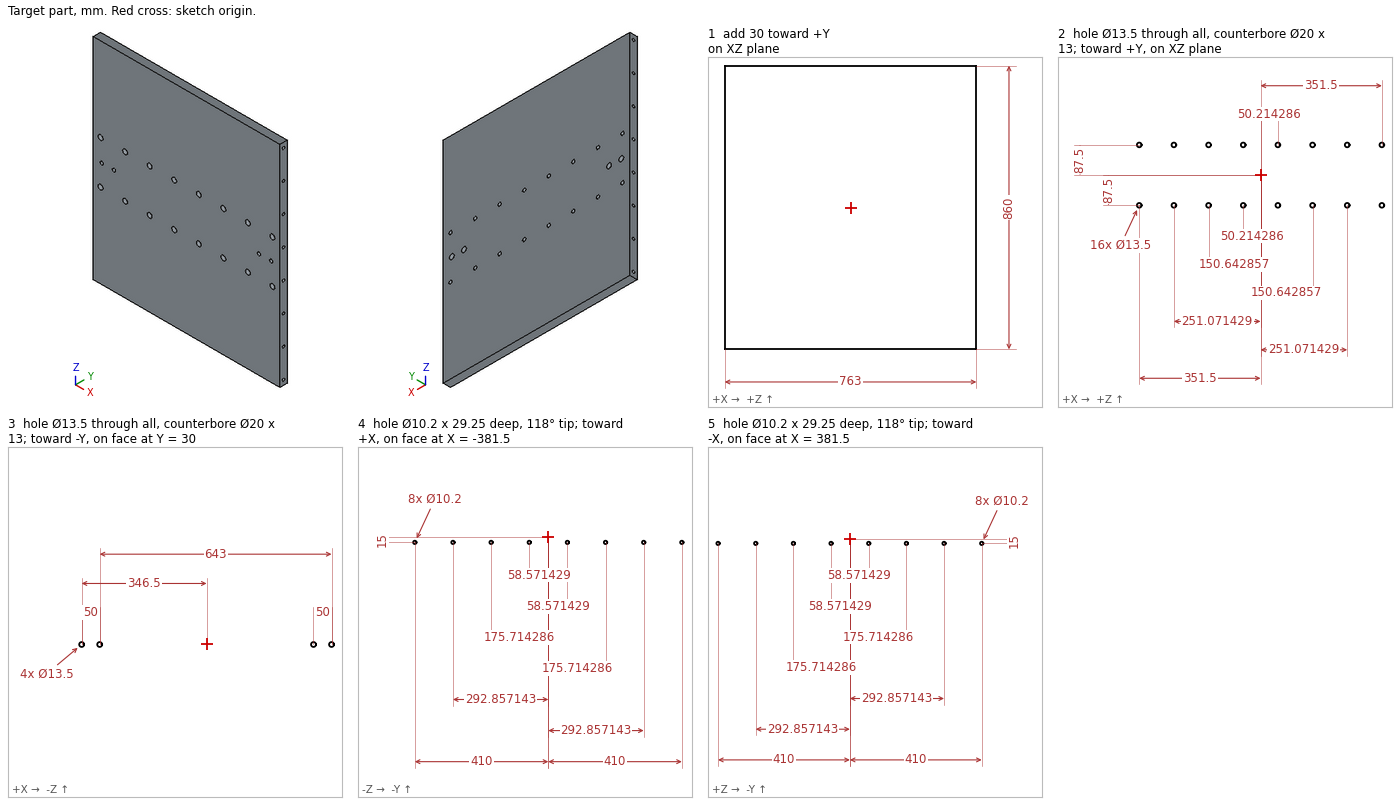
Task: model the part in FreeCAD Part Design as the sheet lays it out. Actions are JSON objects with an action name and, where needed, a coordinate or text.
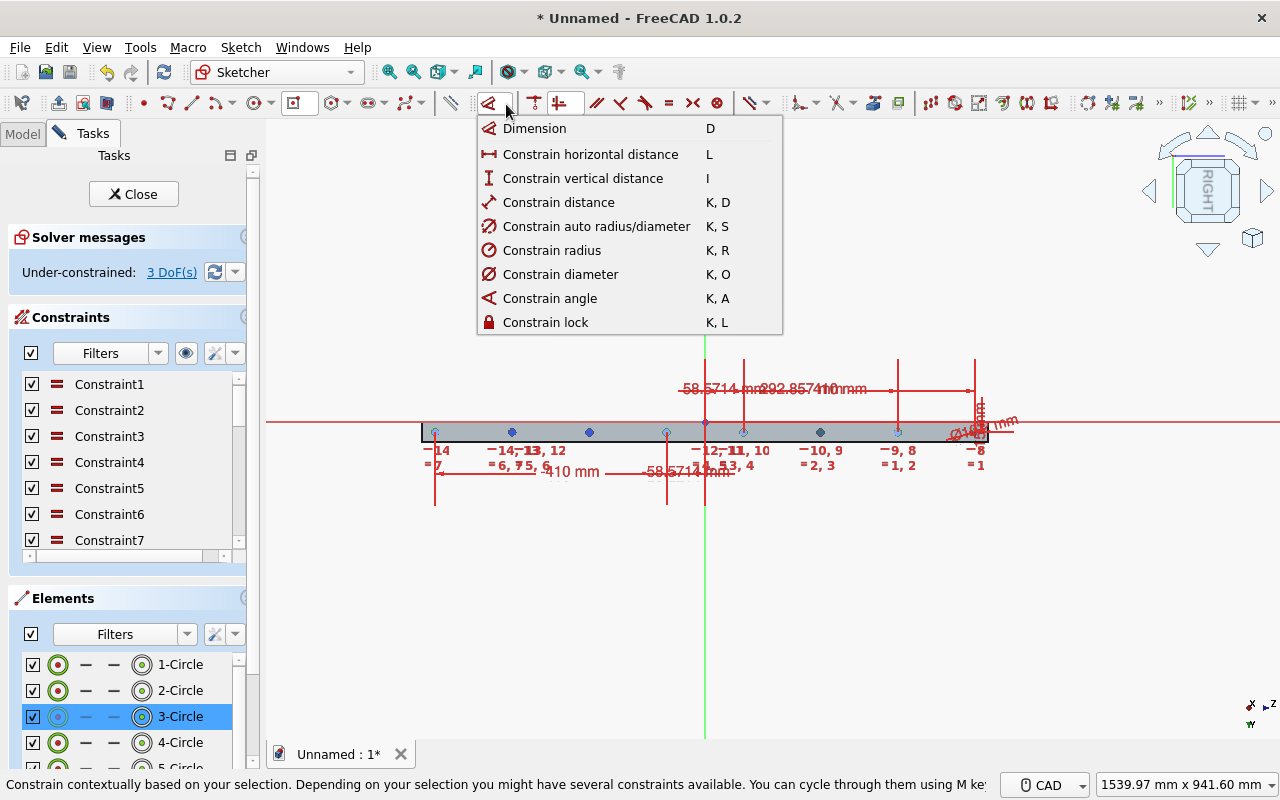
{"action": "left_click", "coordinate": [630, 154]}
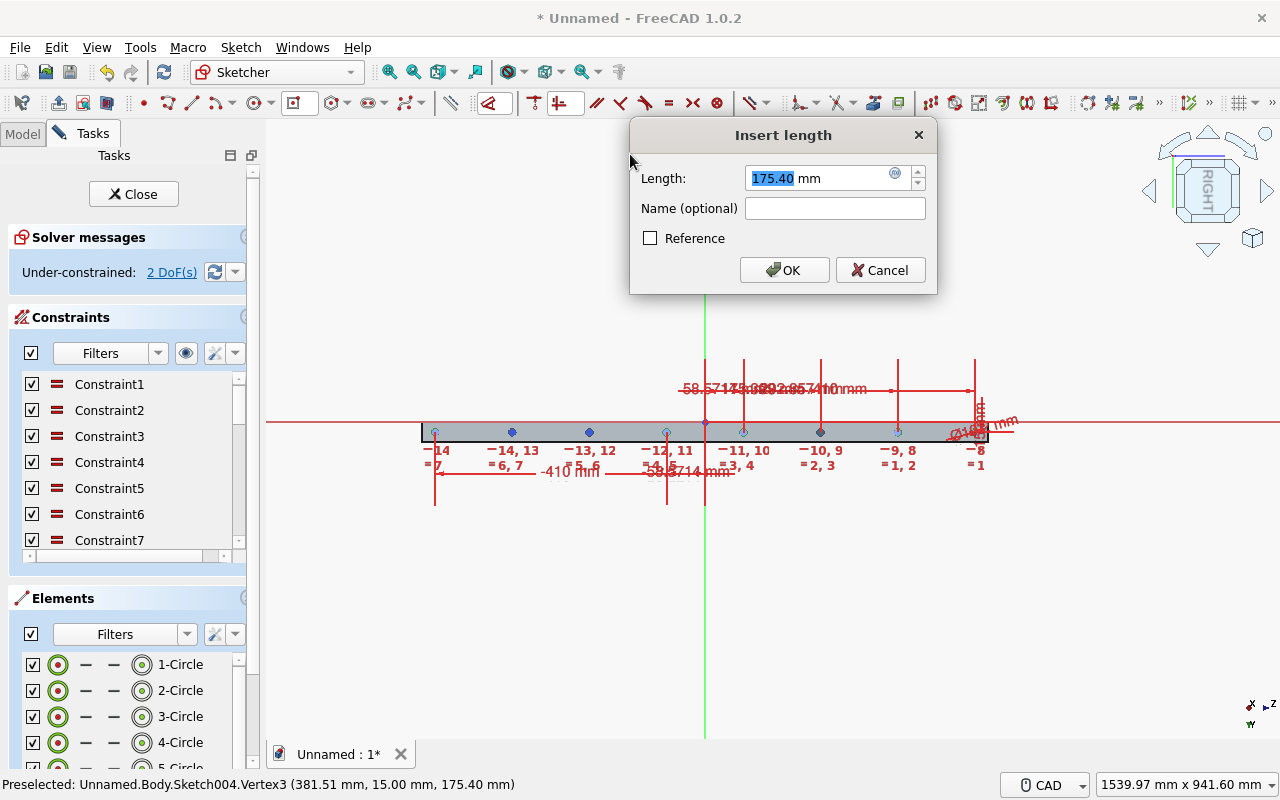
{"action": "type", "text": "175.714286"}
{"action": "key", "text": "Return"}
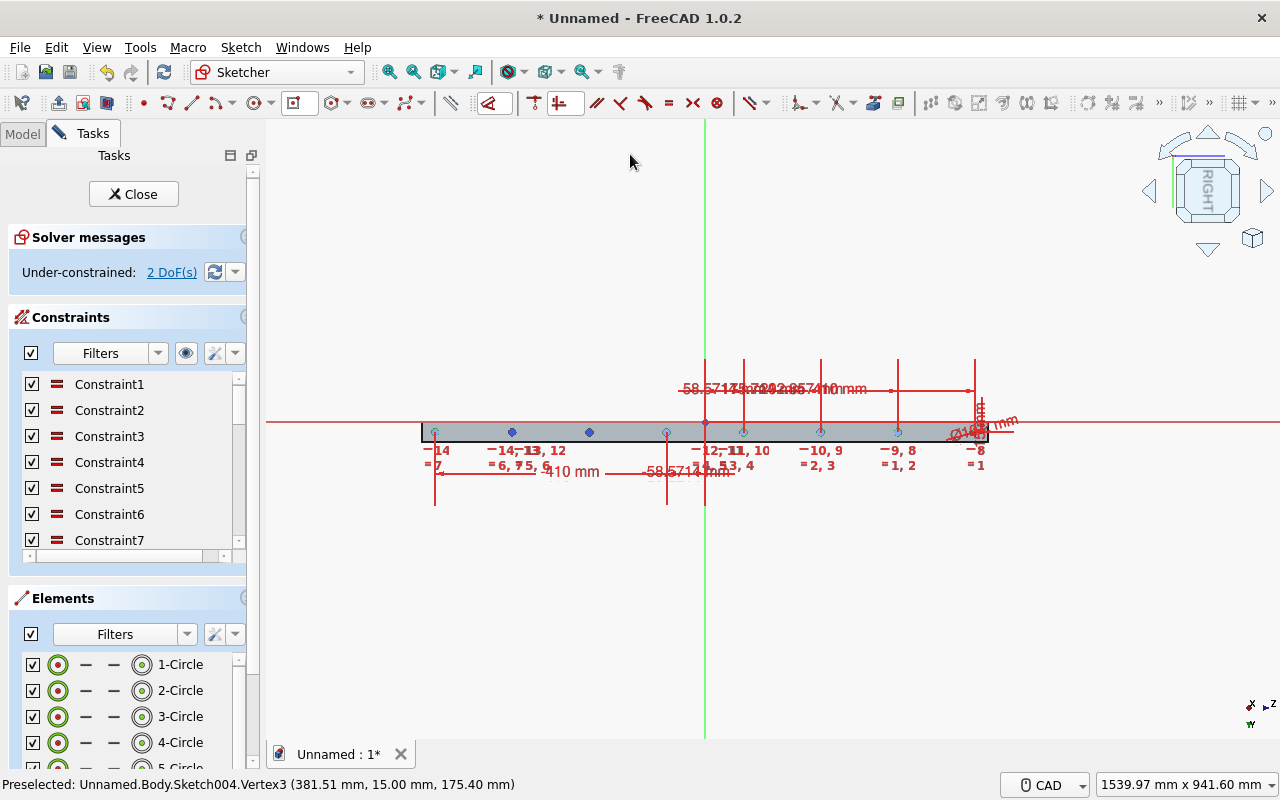
{"action": "left_click", "coordinate": [589, 432]}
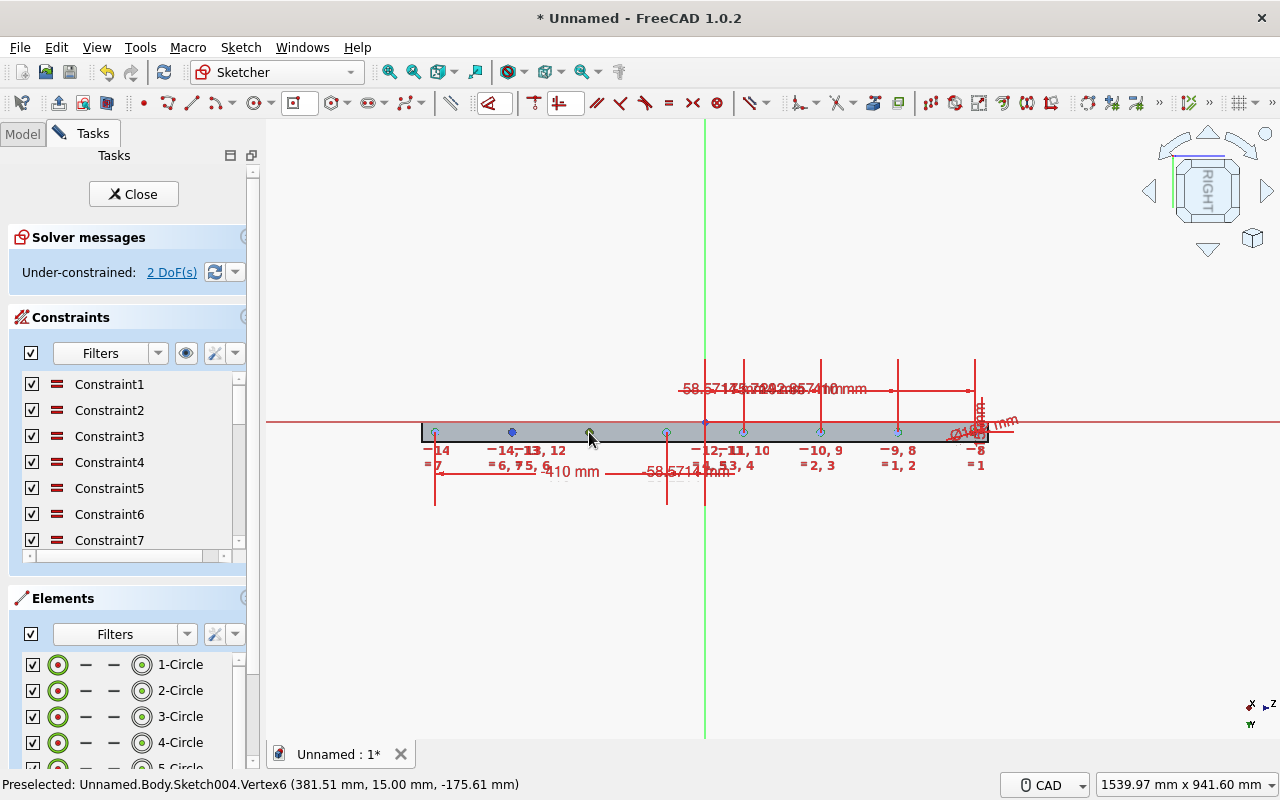
{"action": "left_click", "coordinate": [506, 104]}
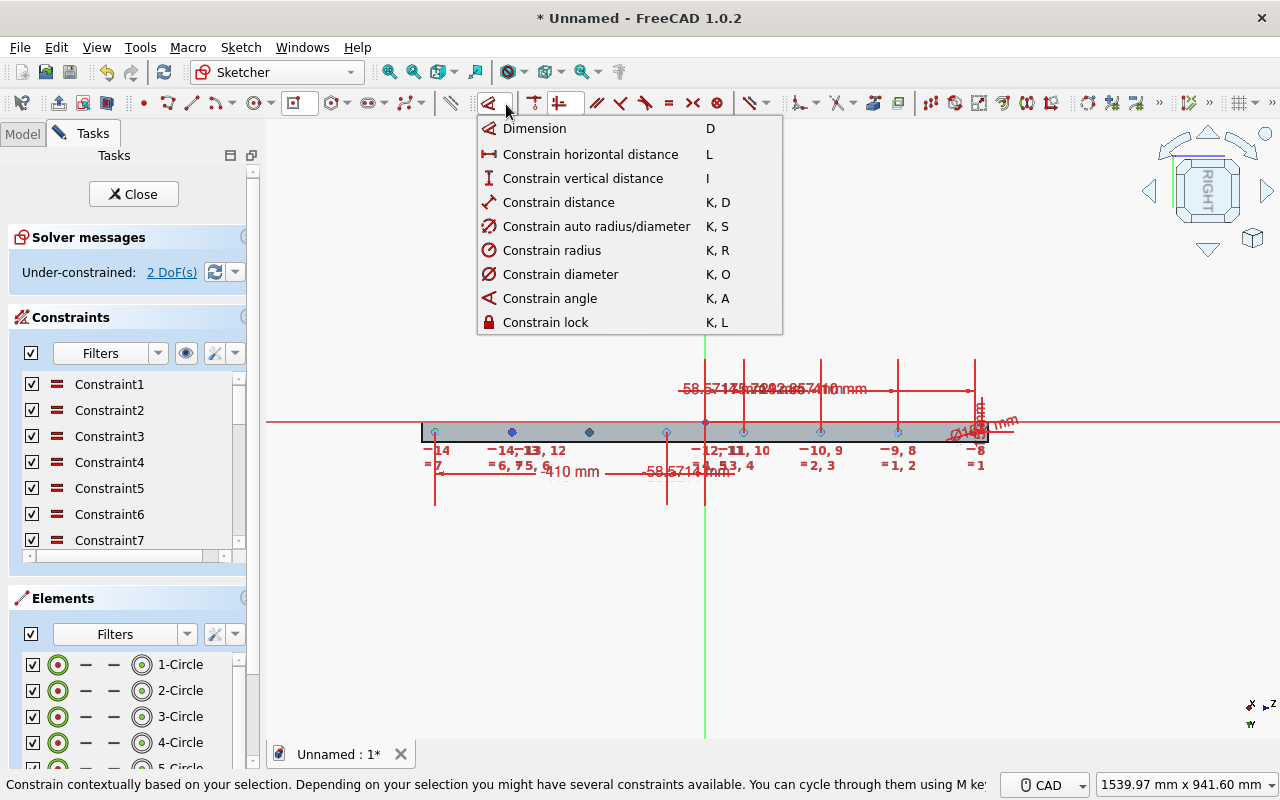
{"action": "left_click", "coordinate": [630, 154]}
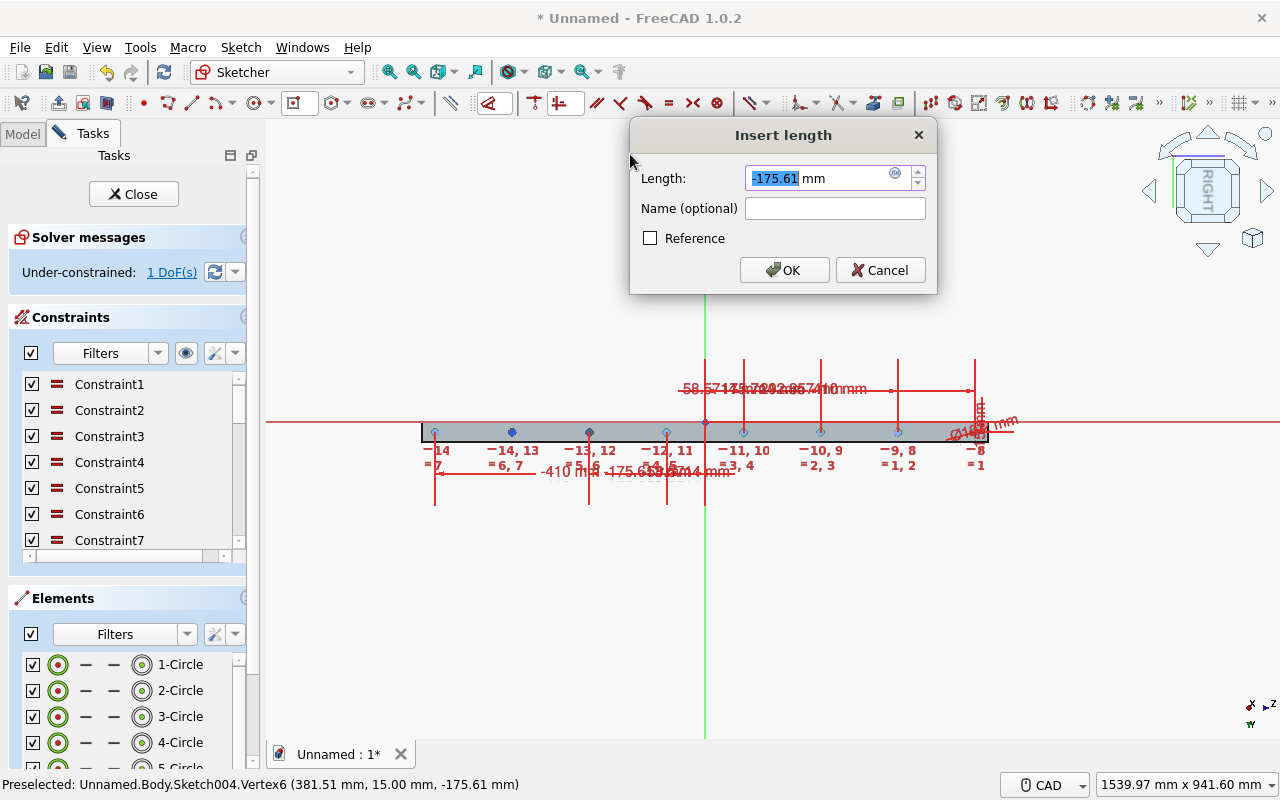
{"action": "type", "text": "-175.714286"}
{"action": "key", "text": "Return"}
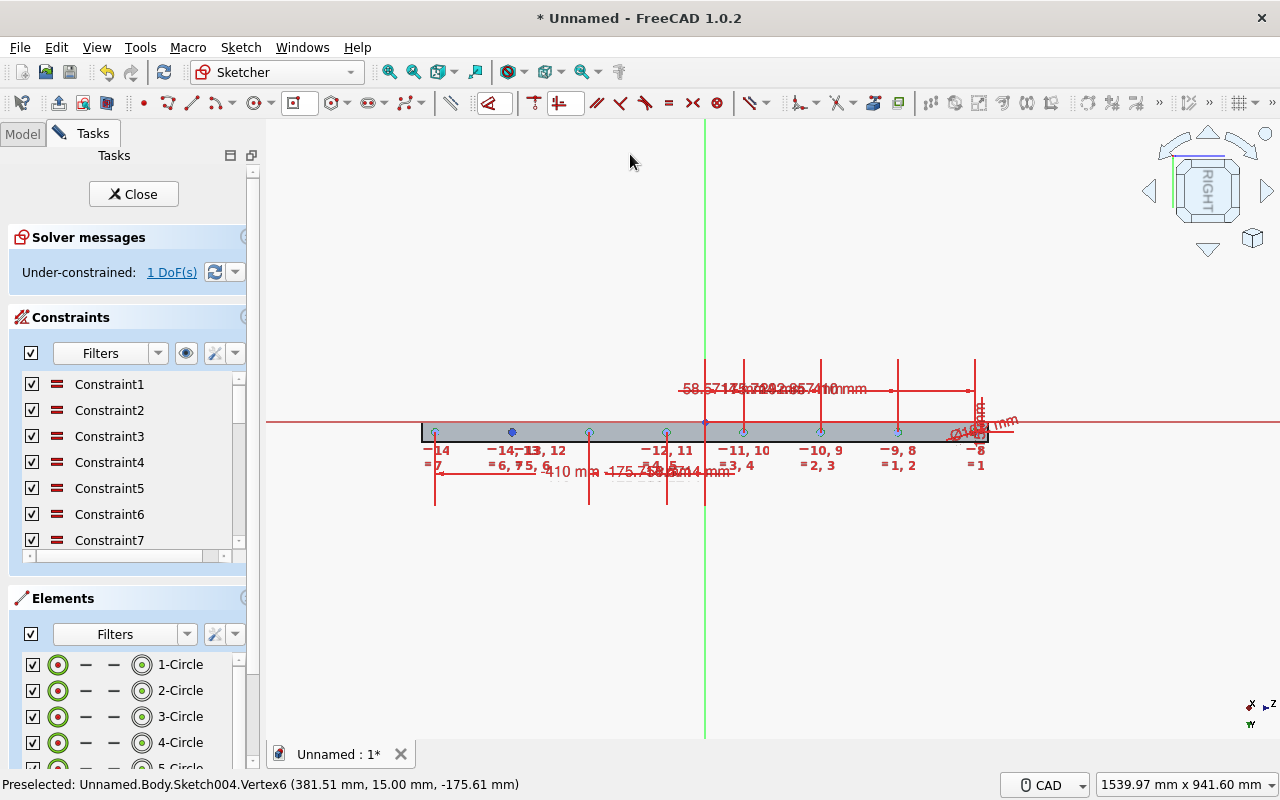
{"action": "left_click", "coordinate": [512, 432]}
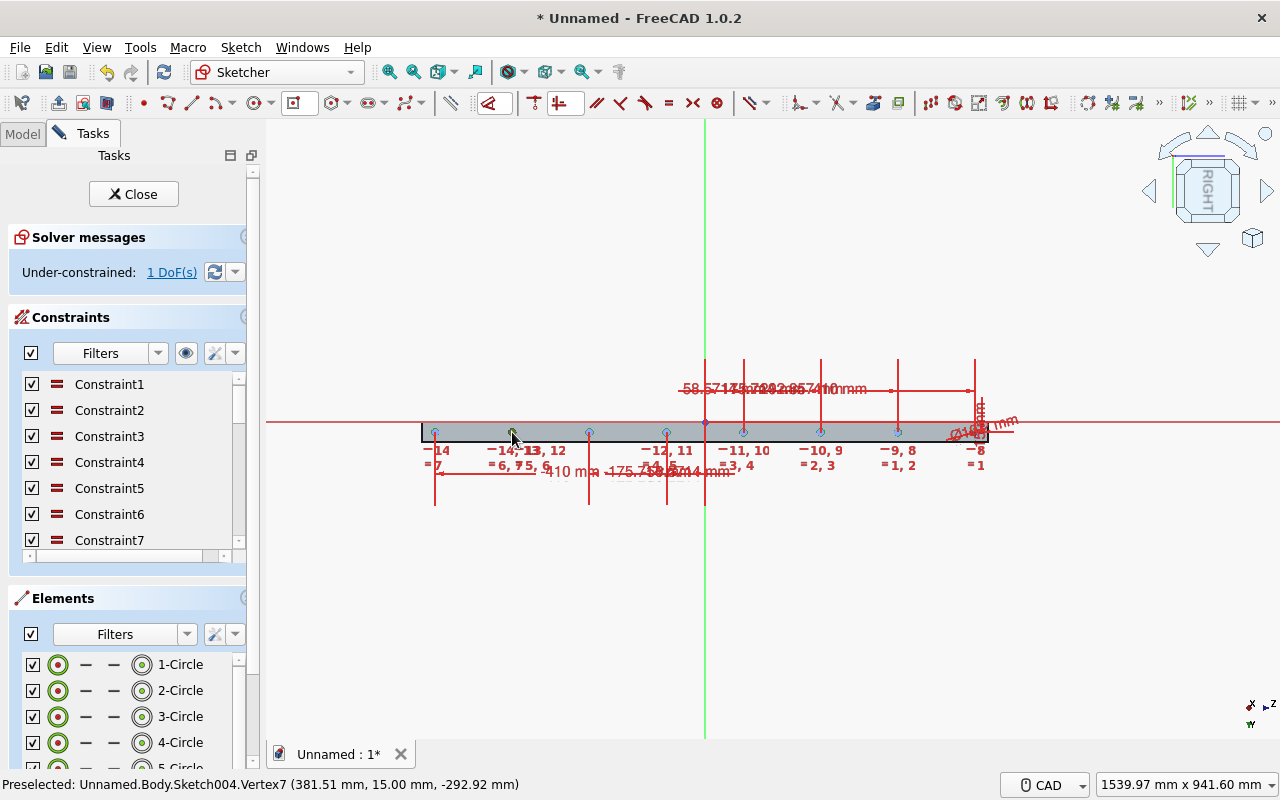
{"action": "key", "text": "l"}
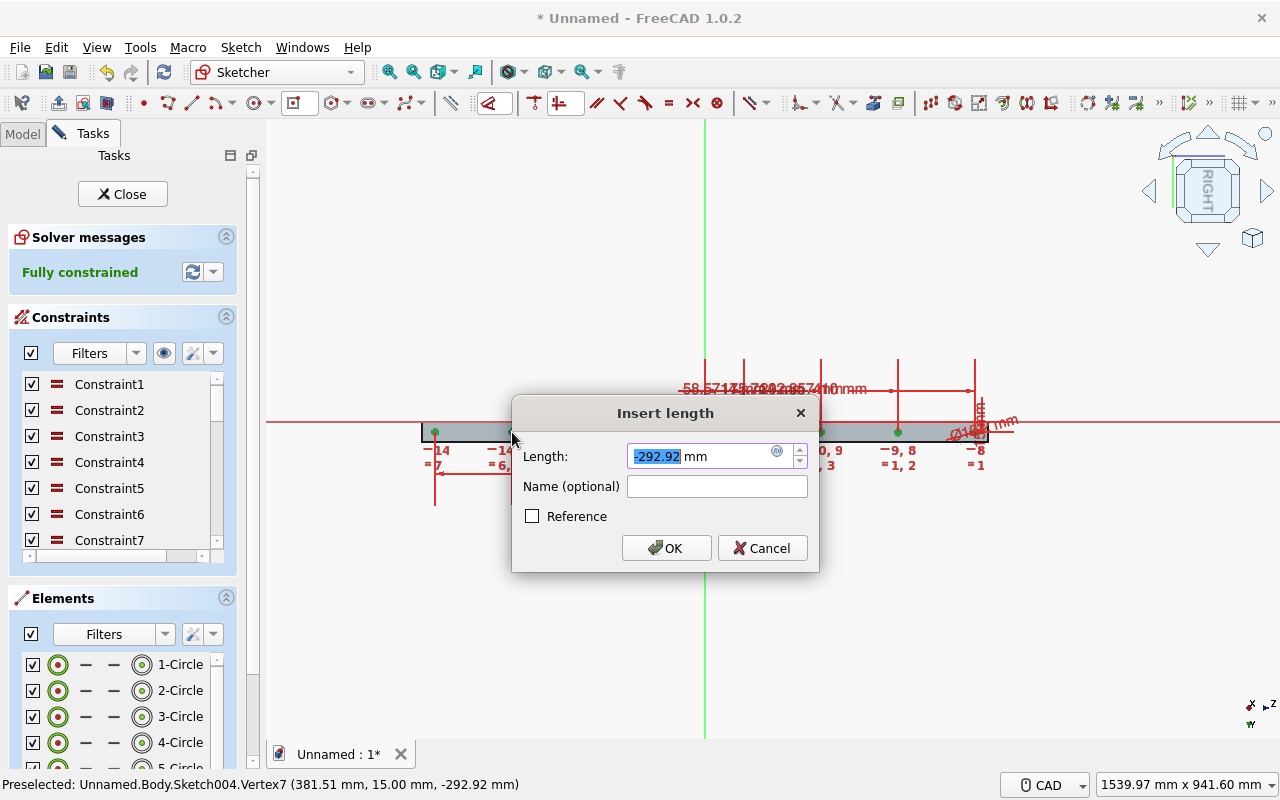
{"action": "type", "text": "-292.857143"}
{"action": "key", "text": "Return"}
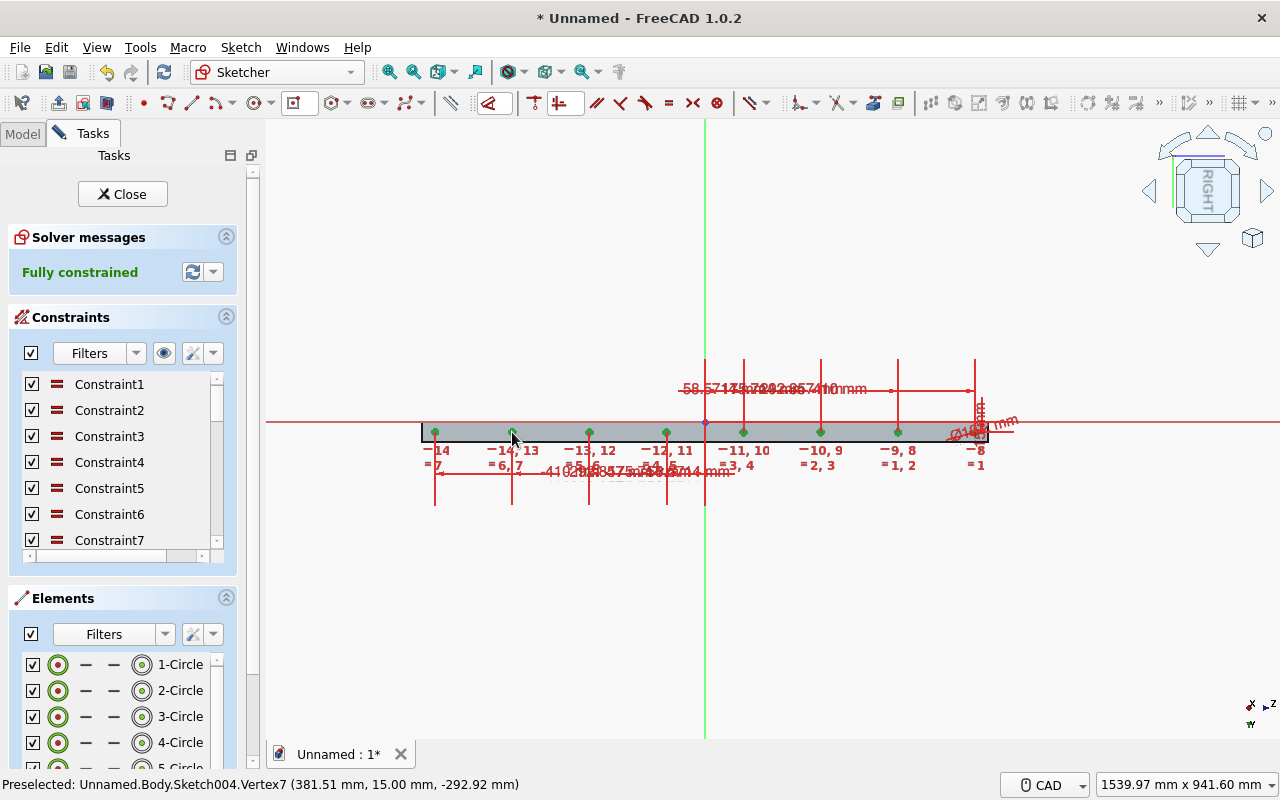
{"action": "left_click", "coordinate": [123, 194]}